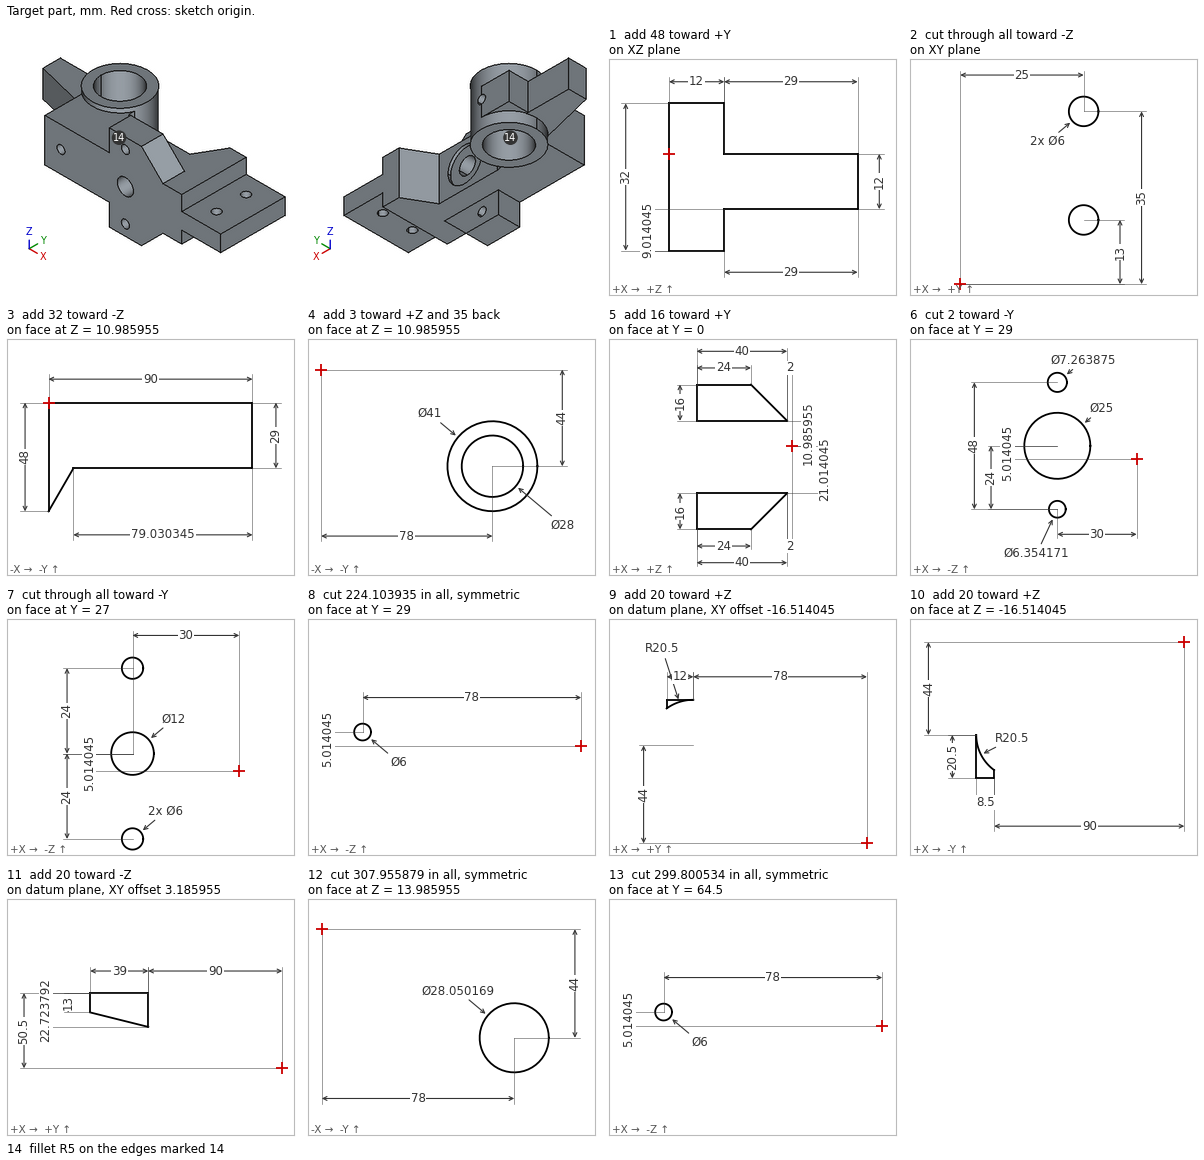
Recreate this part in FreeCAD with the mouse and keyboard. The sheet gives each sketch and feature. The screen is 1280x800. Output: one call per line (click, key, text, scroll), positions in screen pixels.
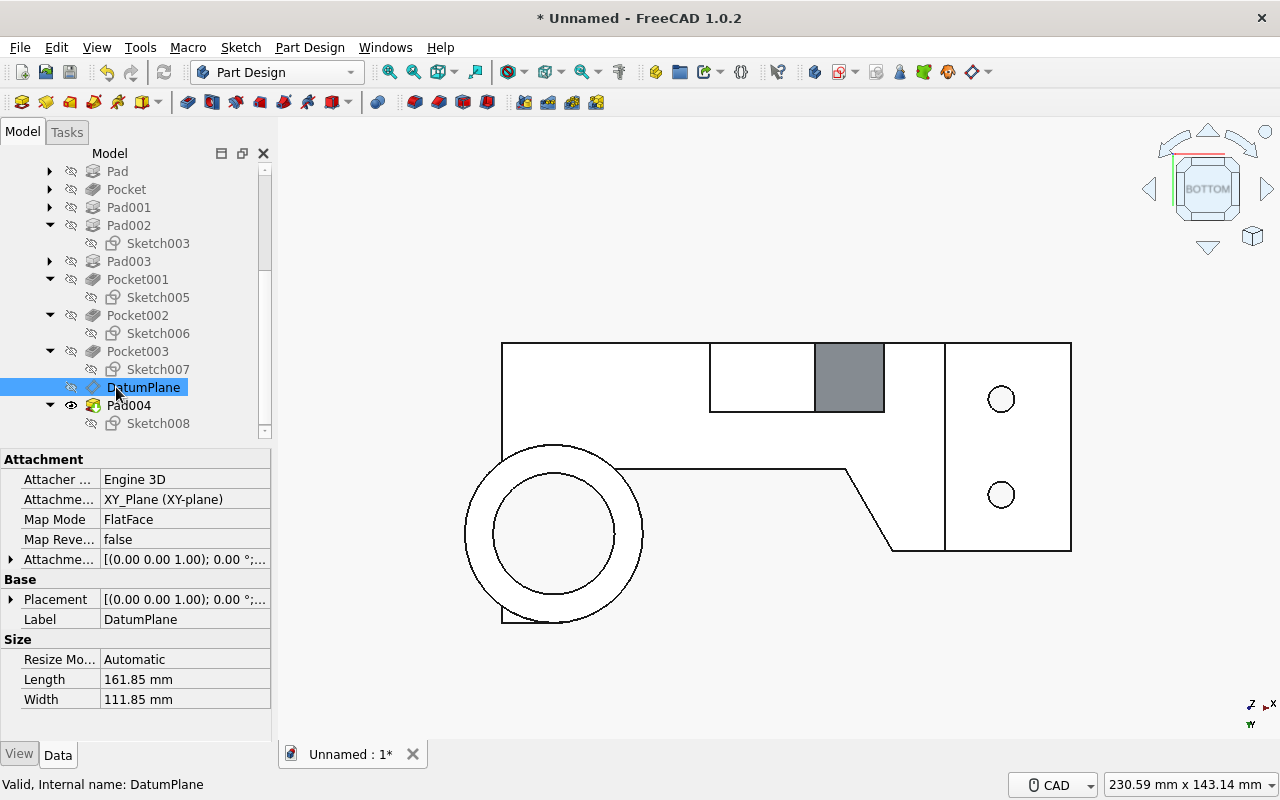
scroll(505, 616, up, 6)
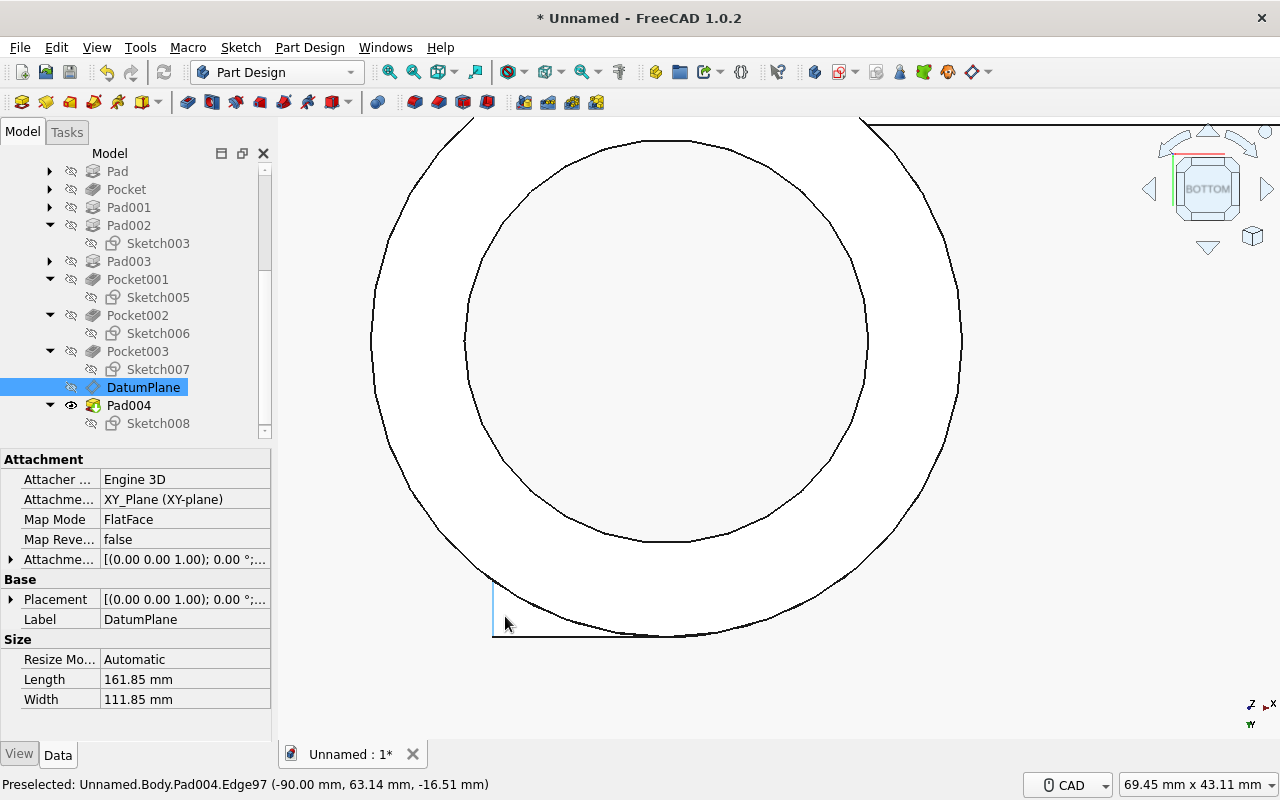
click(506, 616)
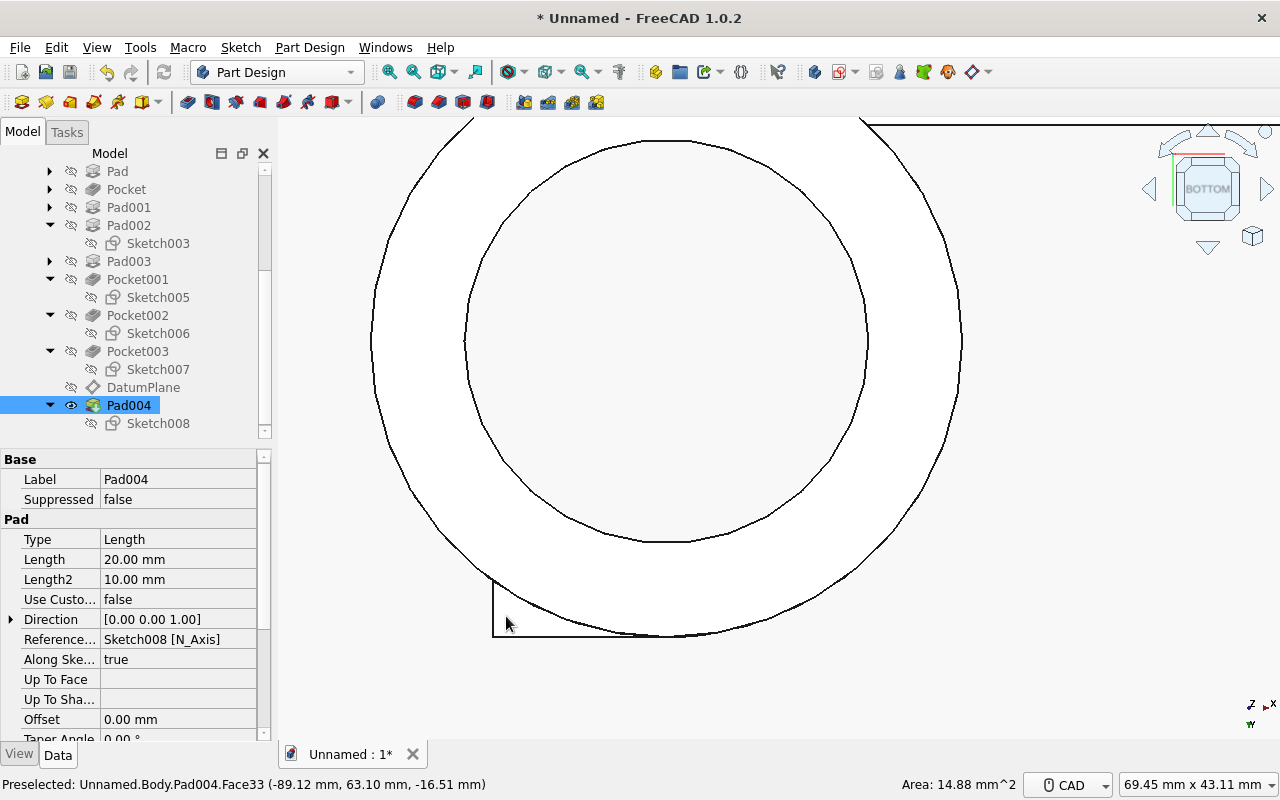
click(840, 72)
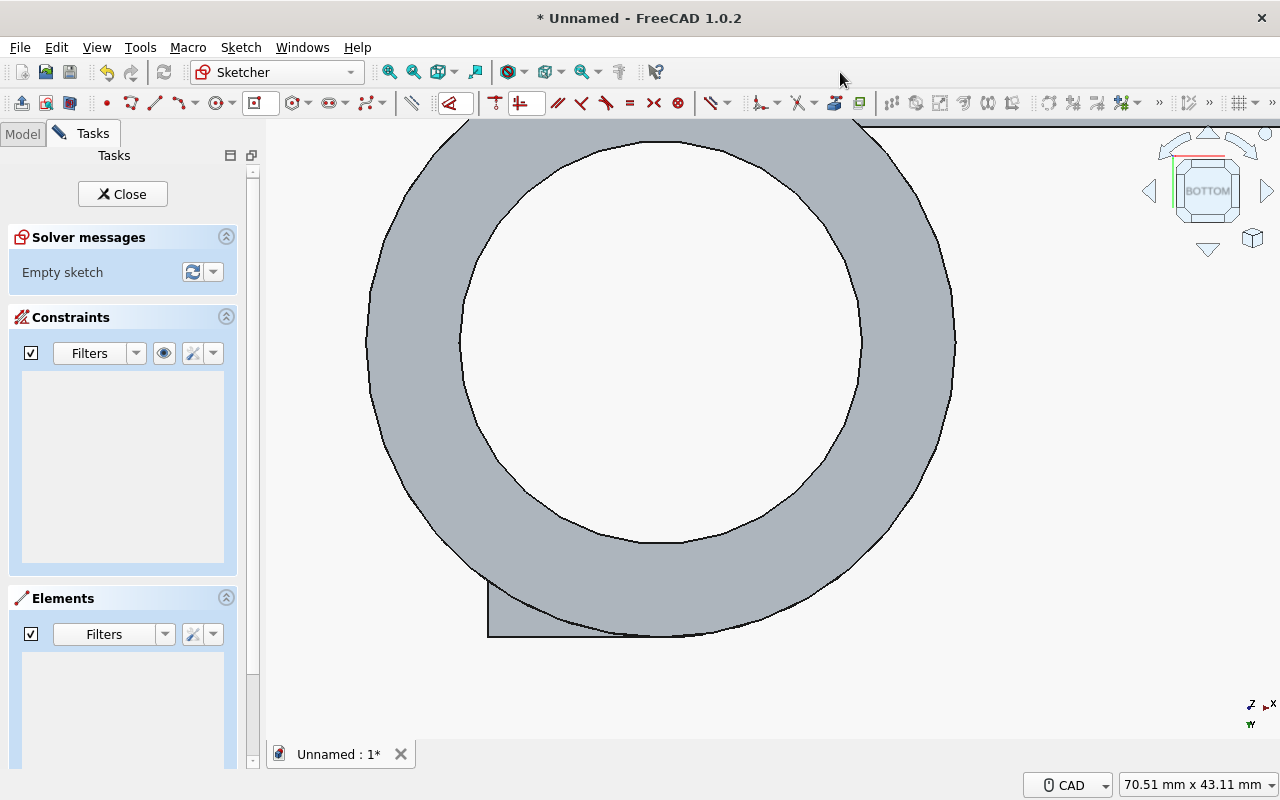
click(70, 104)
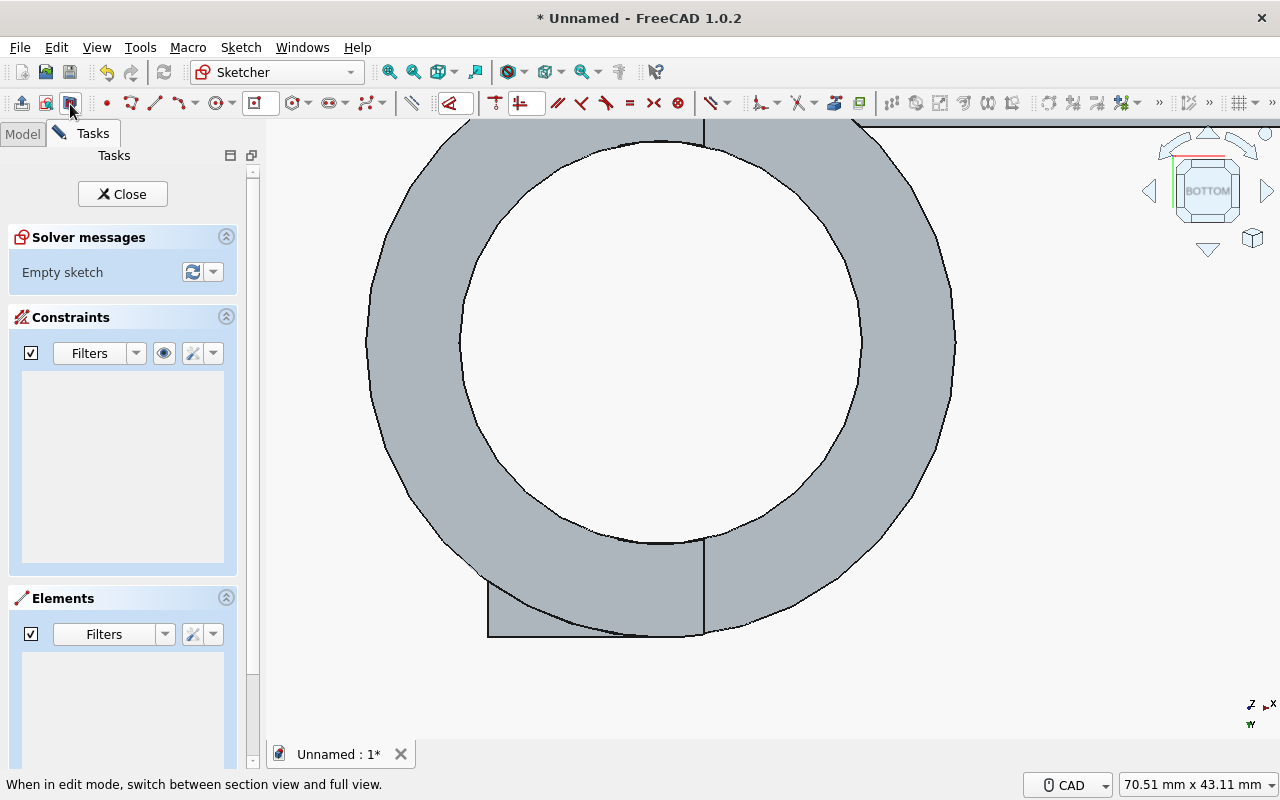
scroll(294, 614, up, 2)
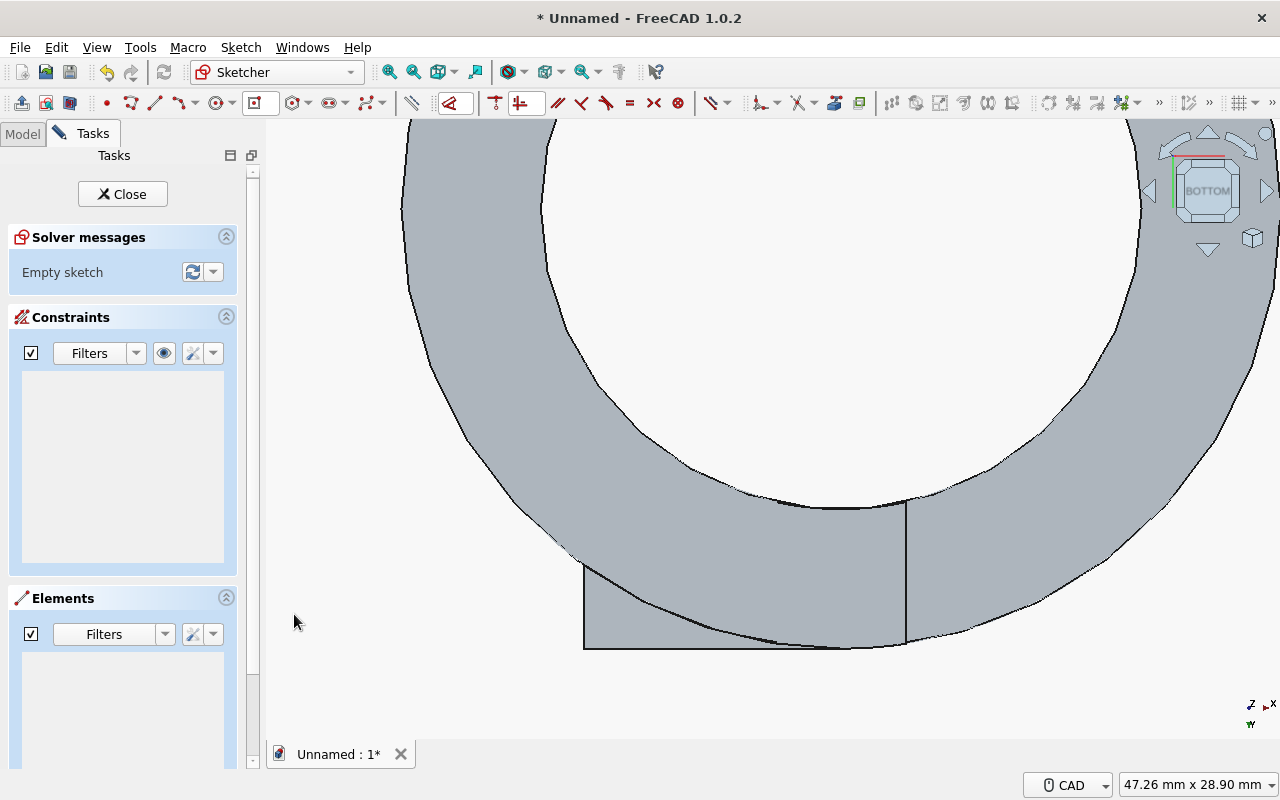
key(g)
key(m)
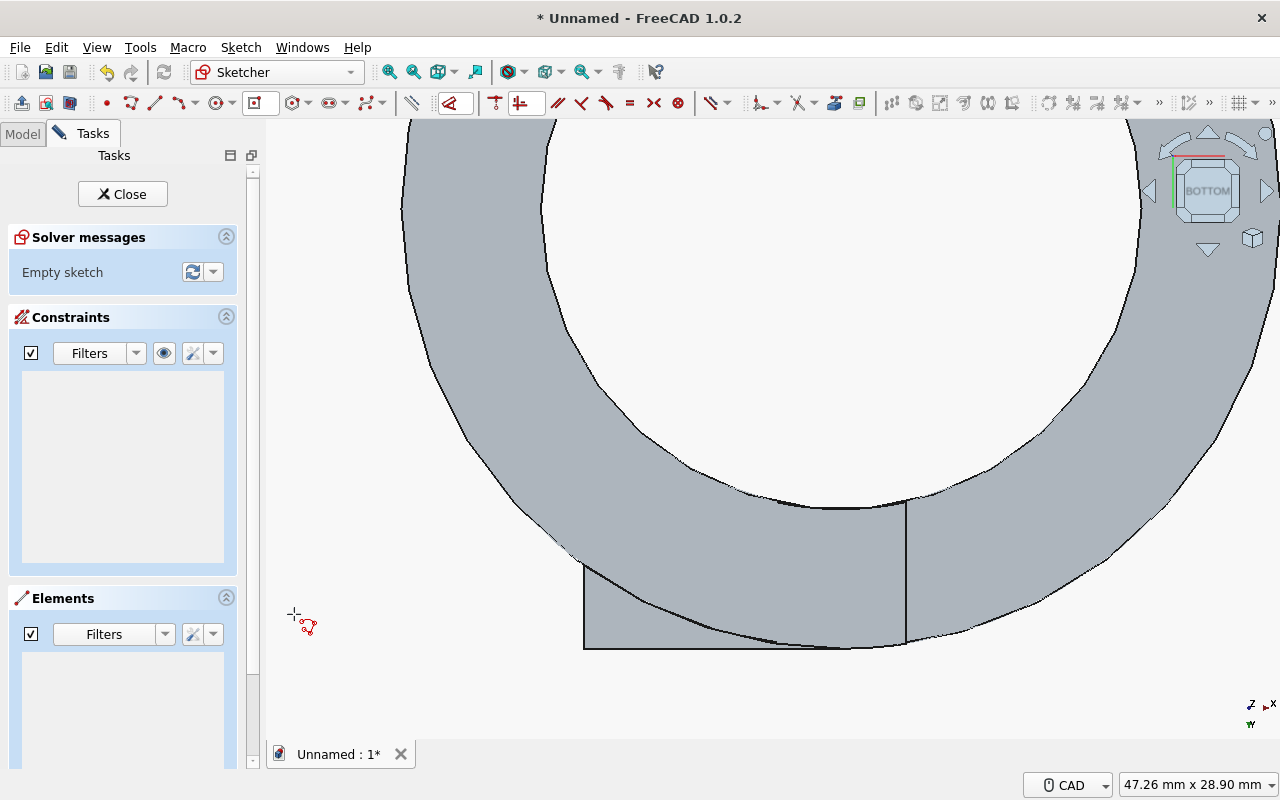
click(584, 565)
click(584, 649)
click(401, 649)
click(401, 209)
right_click(401, 209)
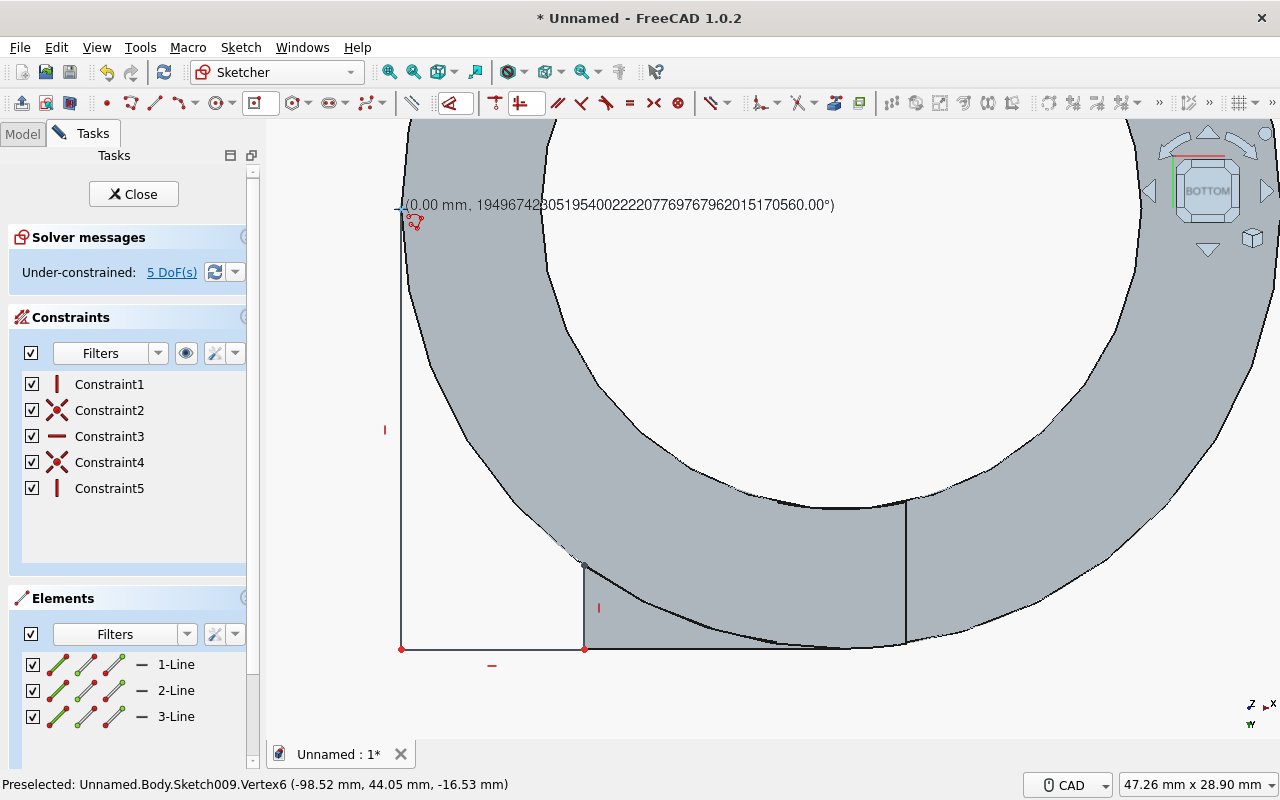
click(180, 104)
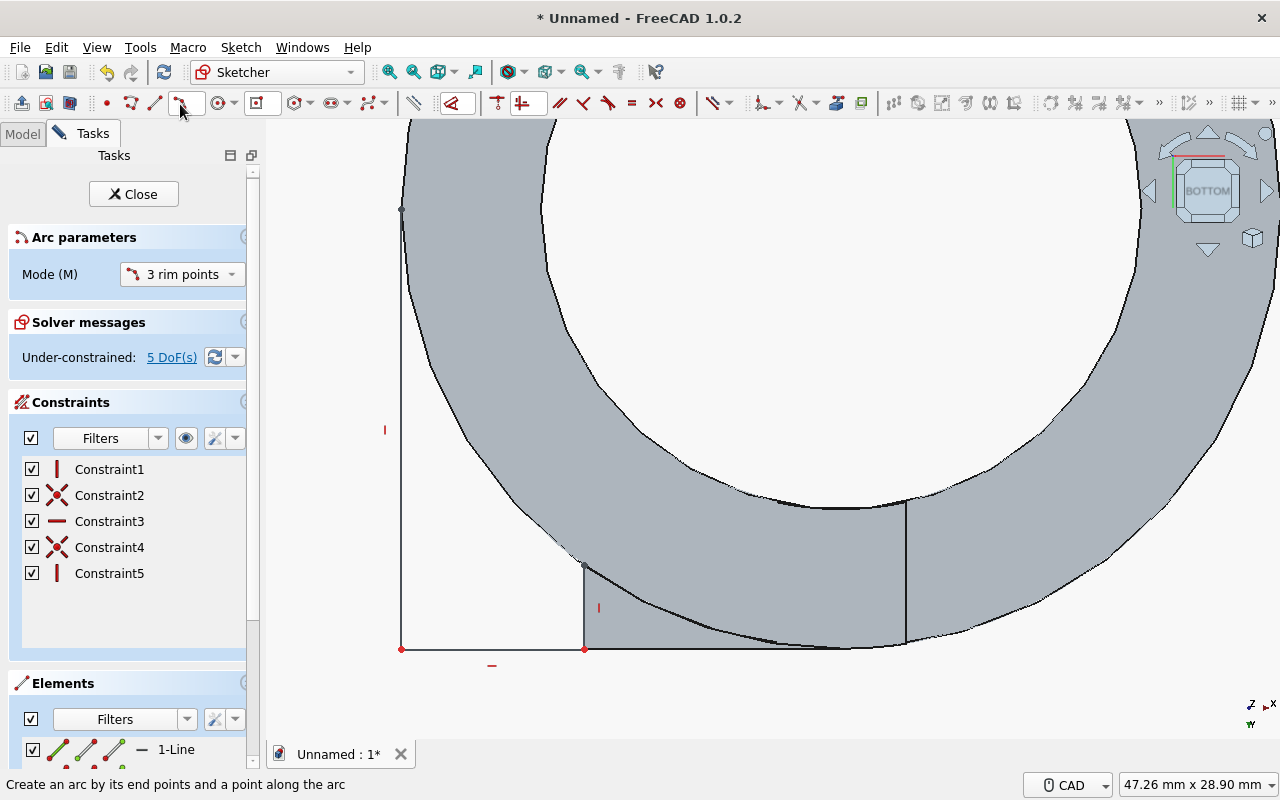
click(401, 210)
click(584, 566)
click(450, 409)
key(Escape)